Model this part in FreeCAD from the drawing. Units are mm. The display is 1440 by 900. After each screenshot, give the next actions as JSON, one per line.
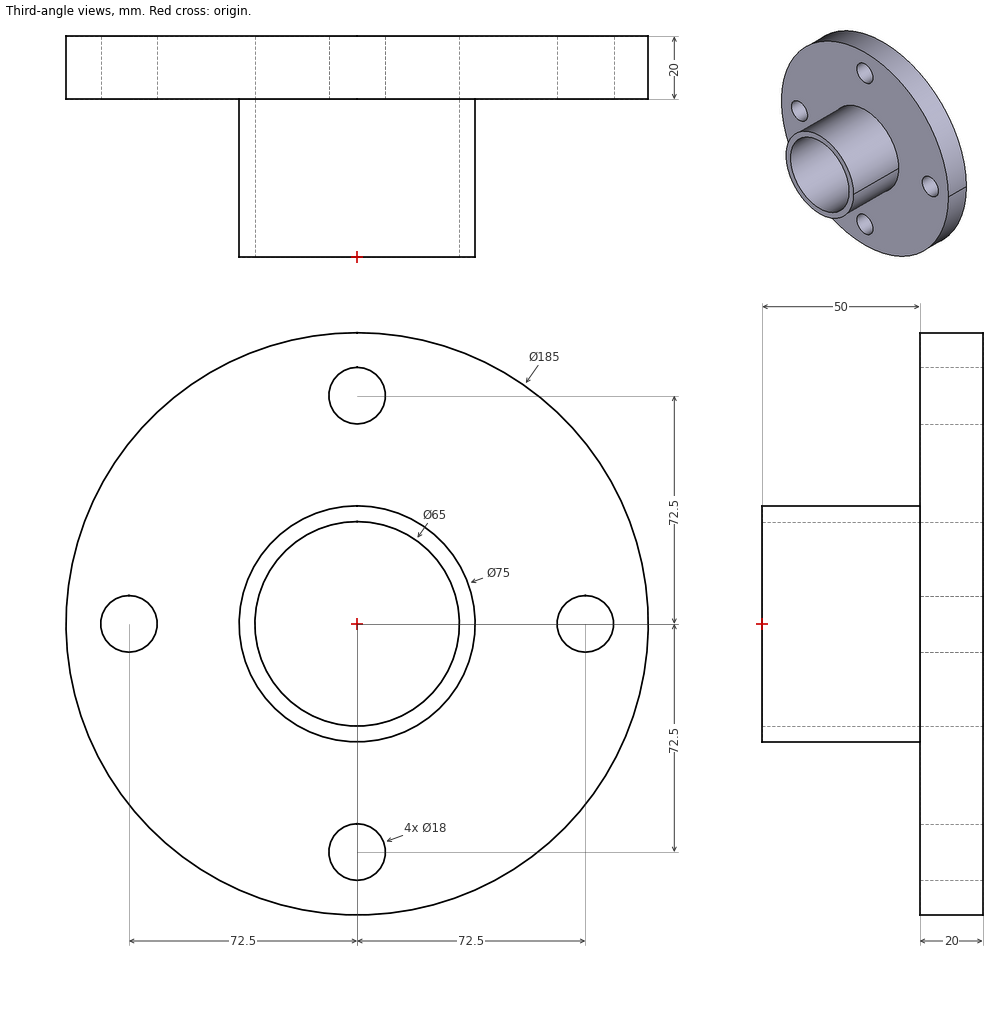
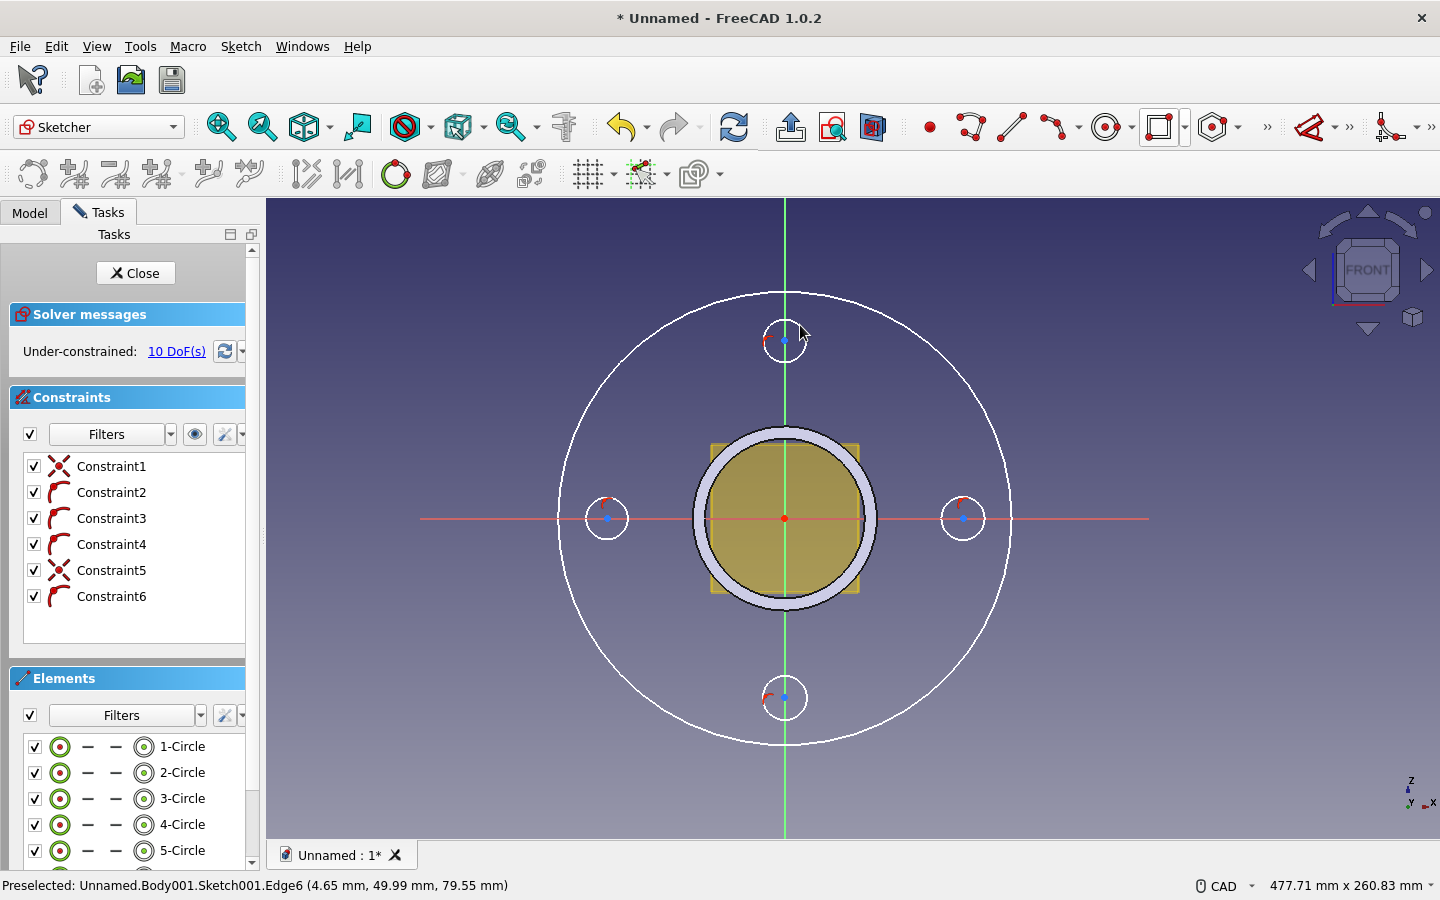
{"action": "left_click", "coordinate": [800, 682]}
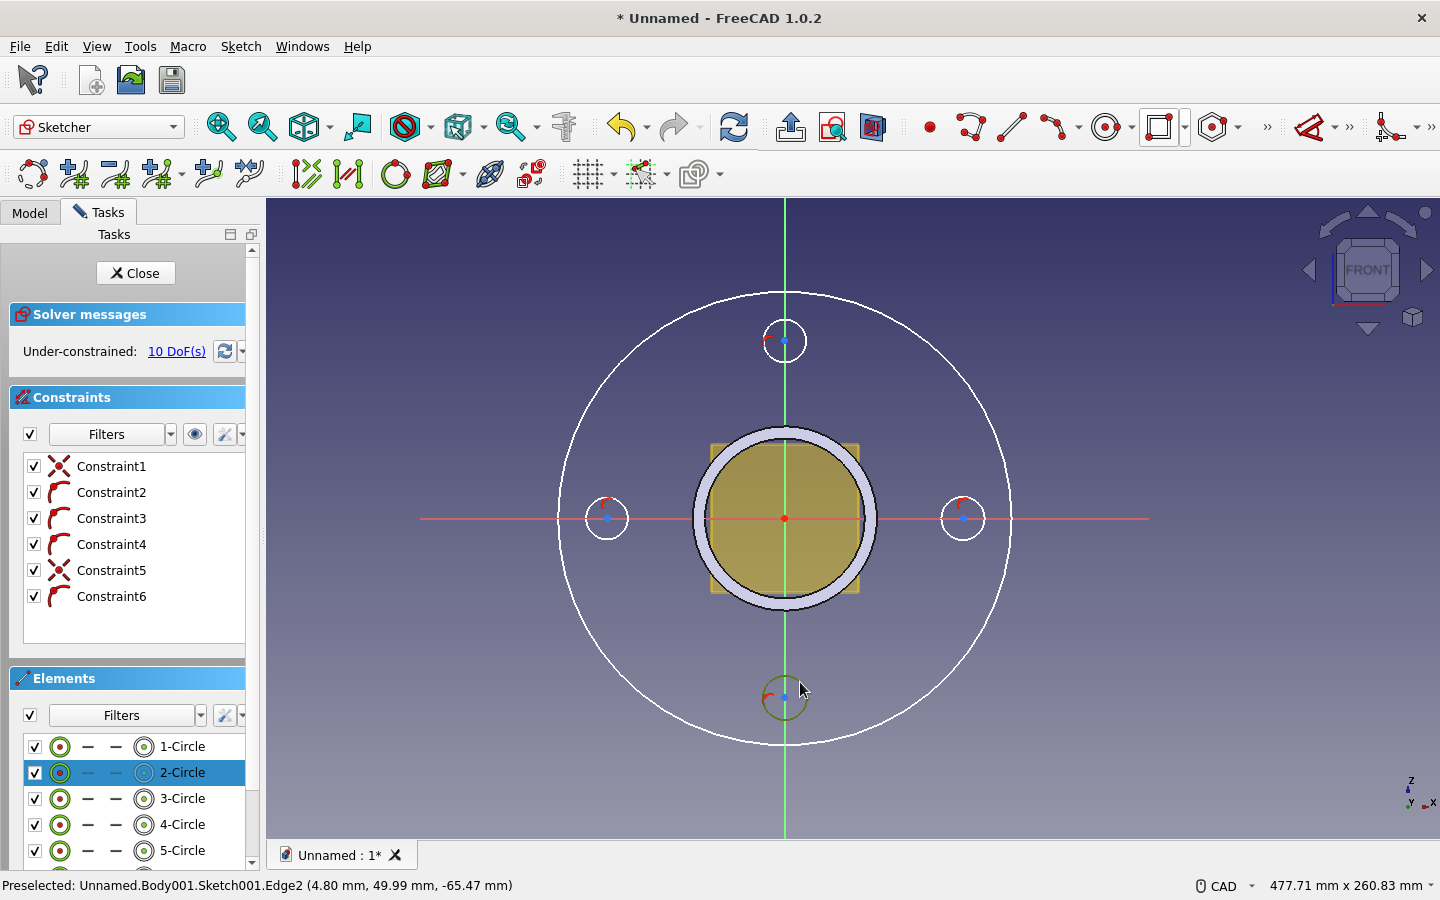
{"action": "left_click", "coordinate": [622, 504]}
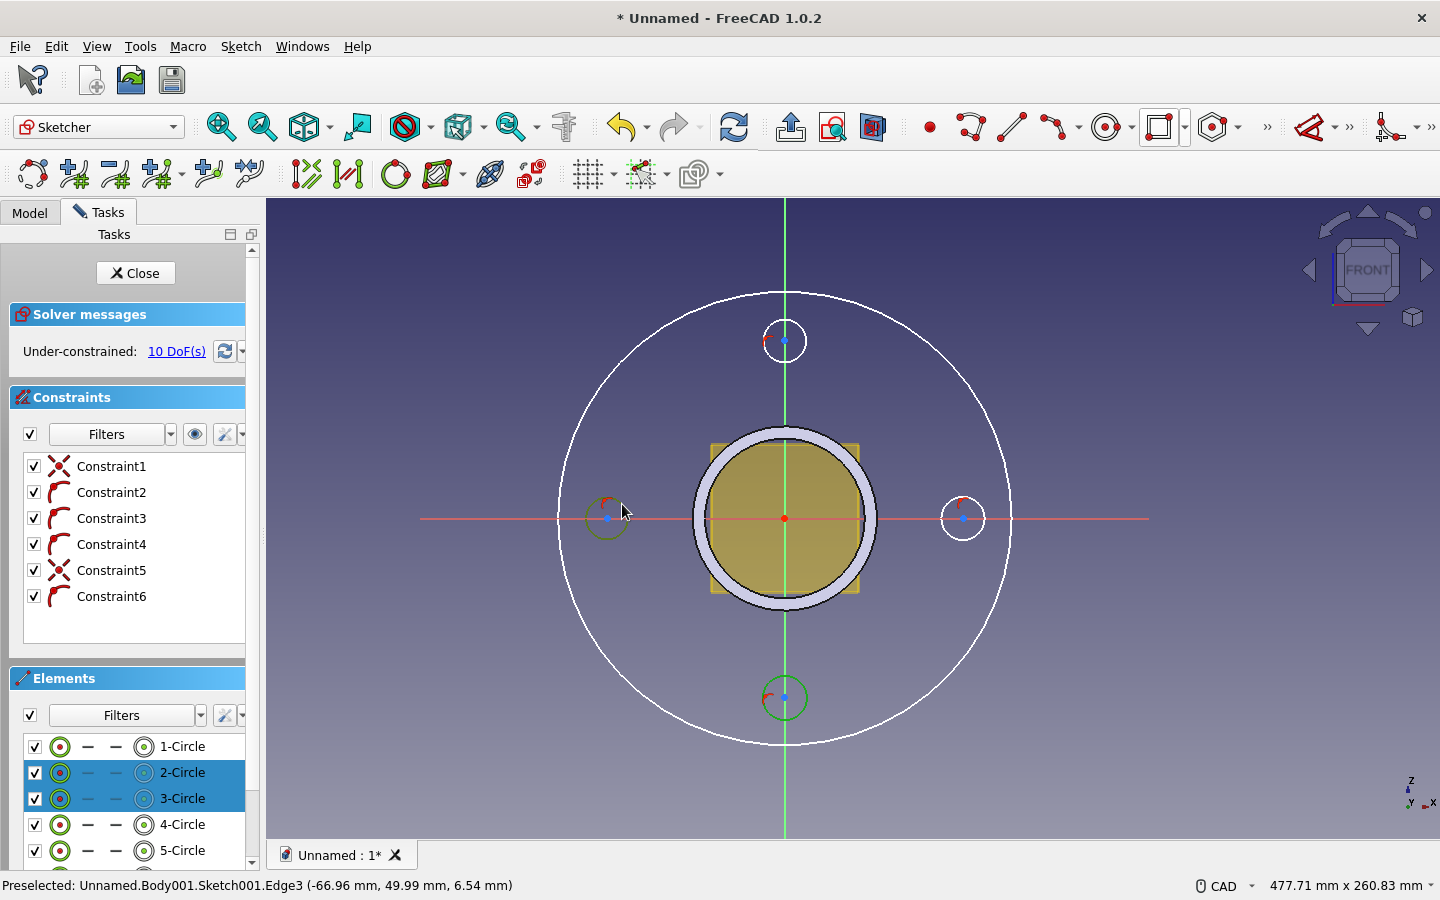
{"action": "left_click", "coordinate": [978, 503]}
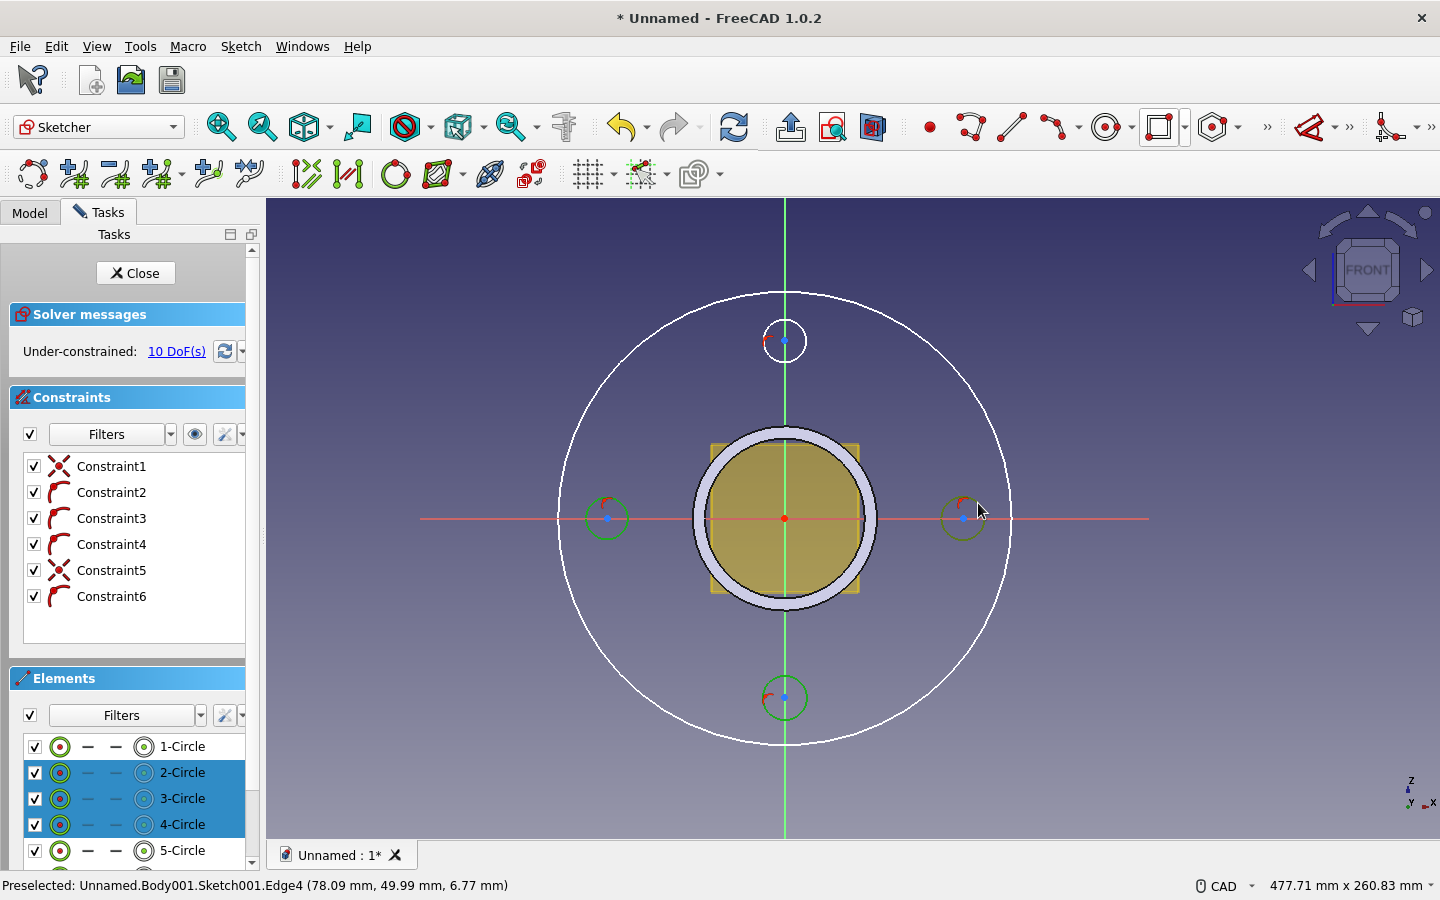
{"action": "left_click", "coordinate": [800, 326]}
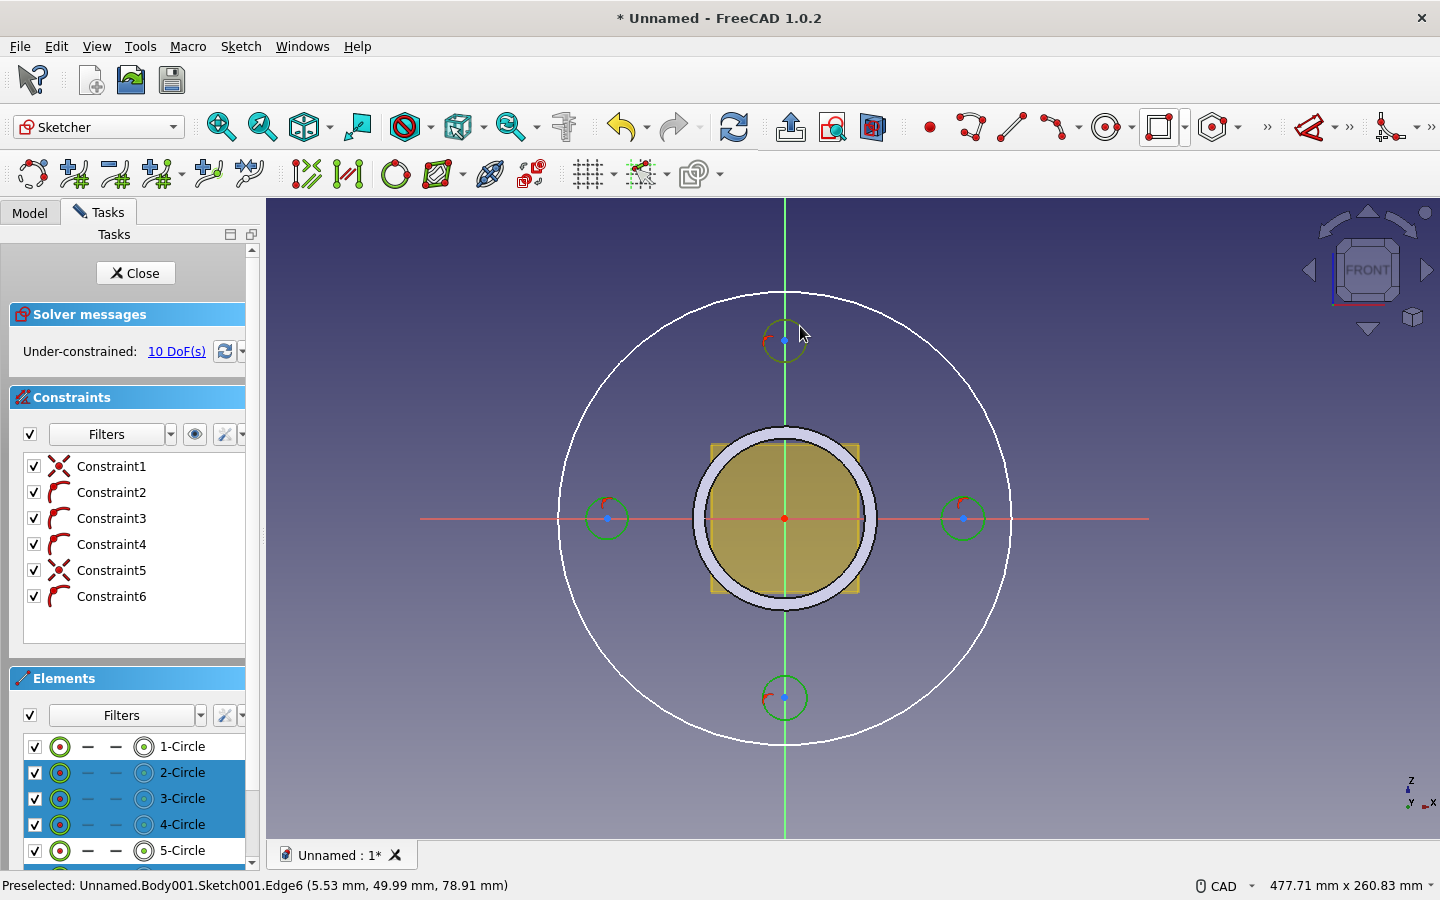
{"action": "key", "text": "e"}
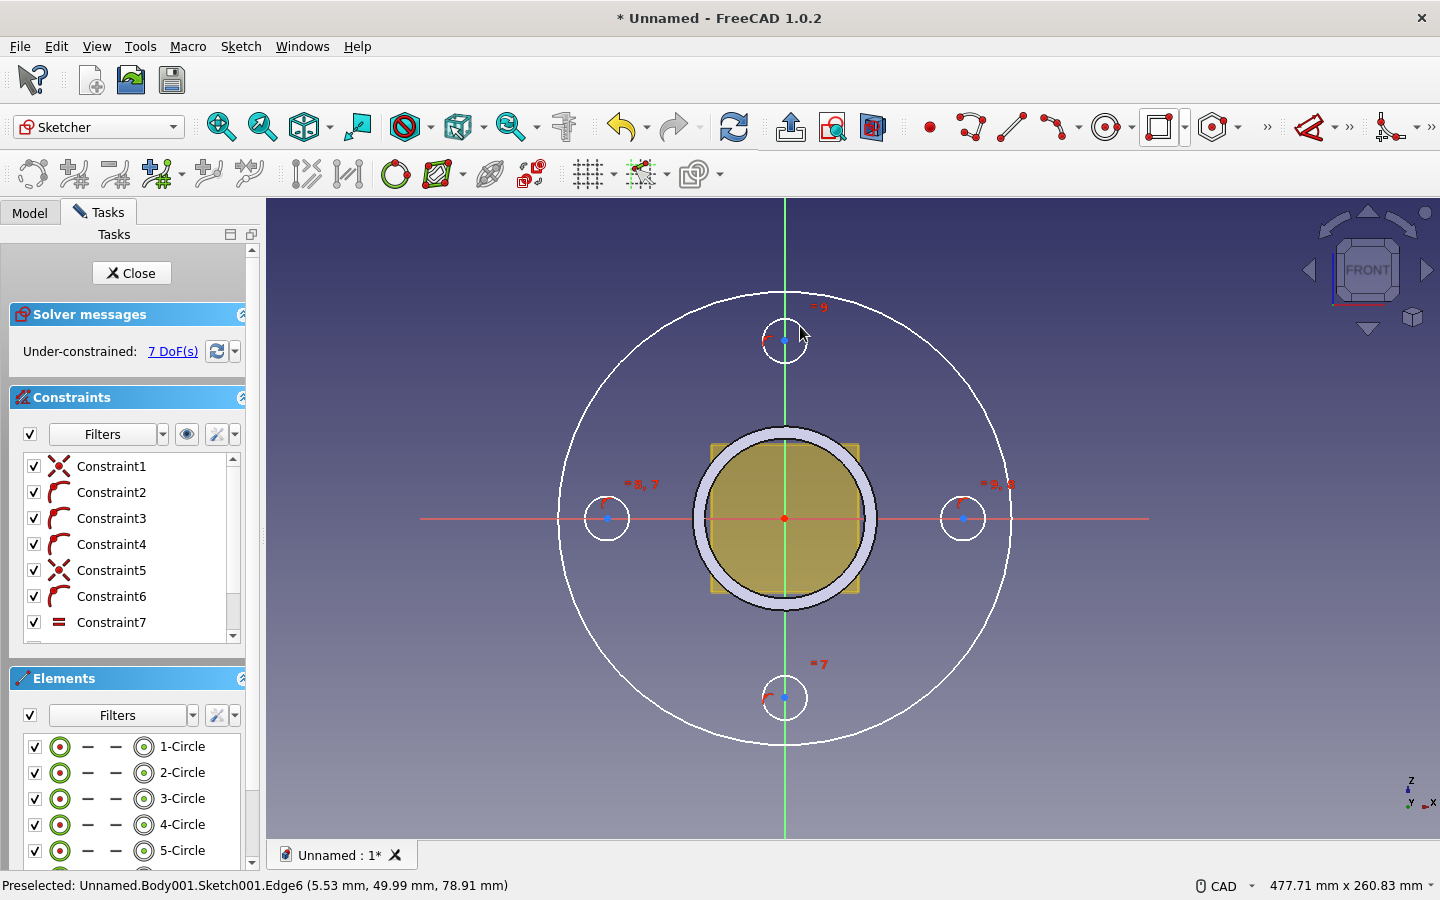
{"action": "key", "text": "d"}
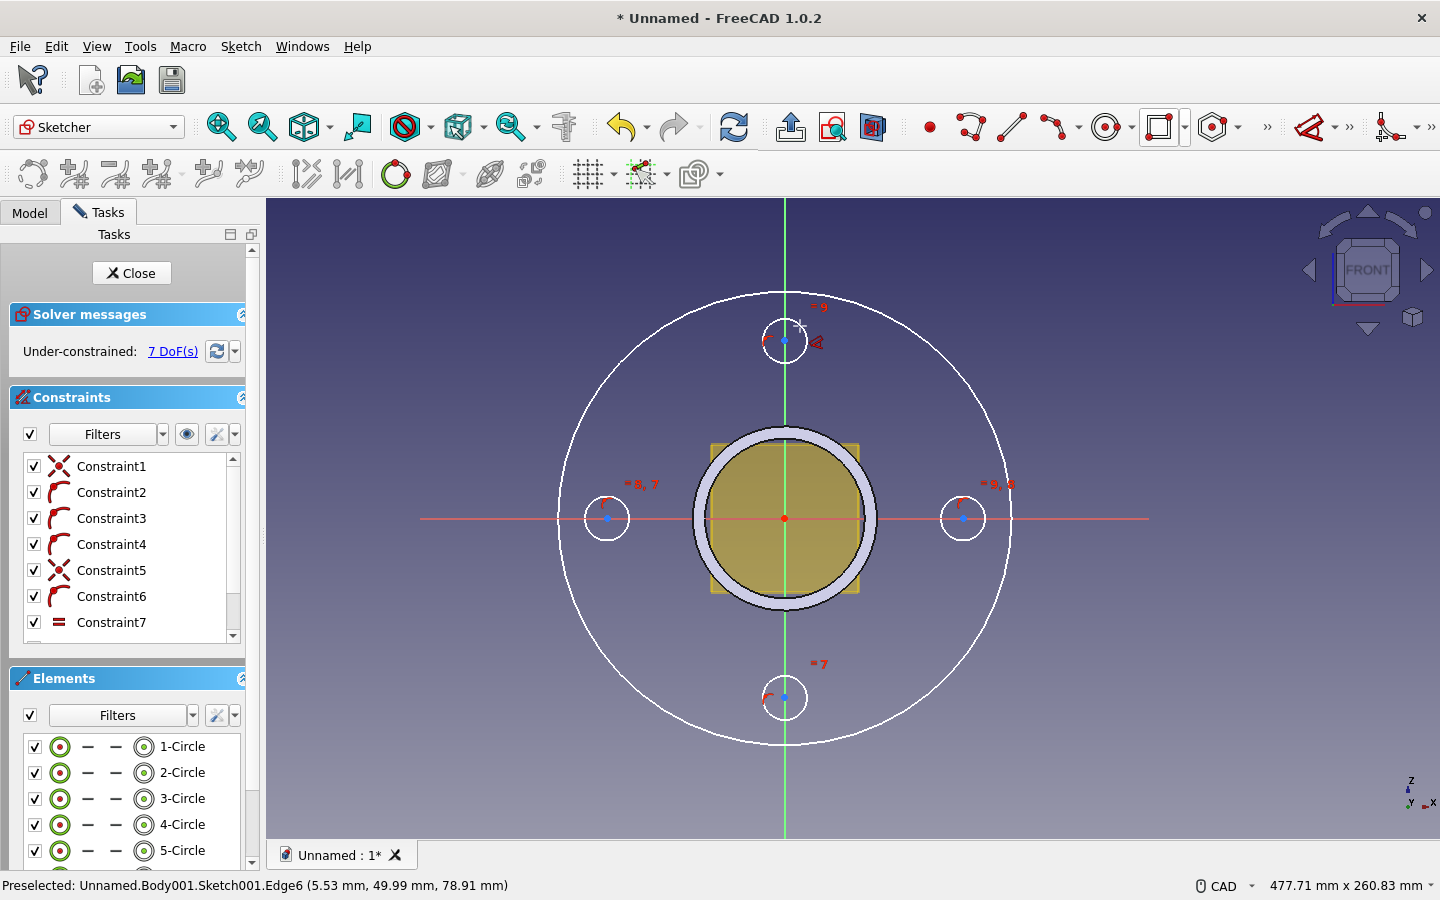
{"action": "left_click", "coordinate": [945, 358]}
{"action": "left_click", "coordinate": [968, 335]}